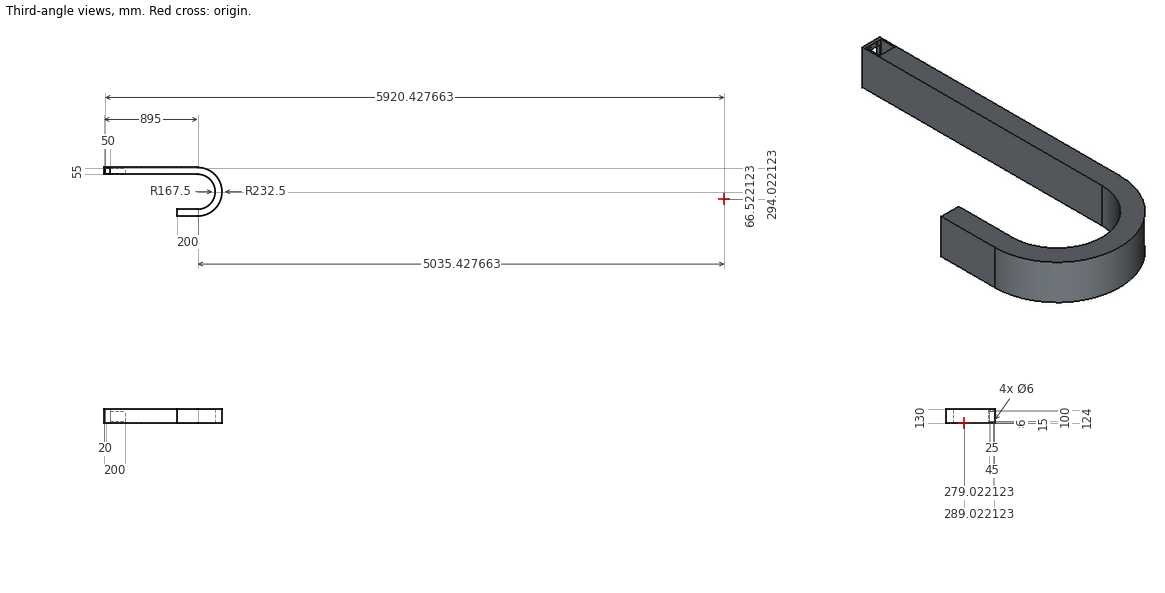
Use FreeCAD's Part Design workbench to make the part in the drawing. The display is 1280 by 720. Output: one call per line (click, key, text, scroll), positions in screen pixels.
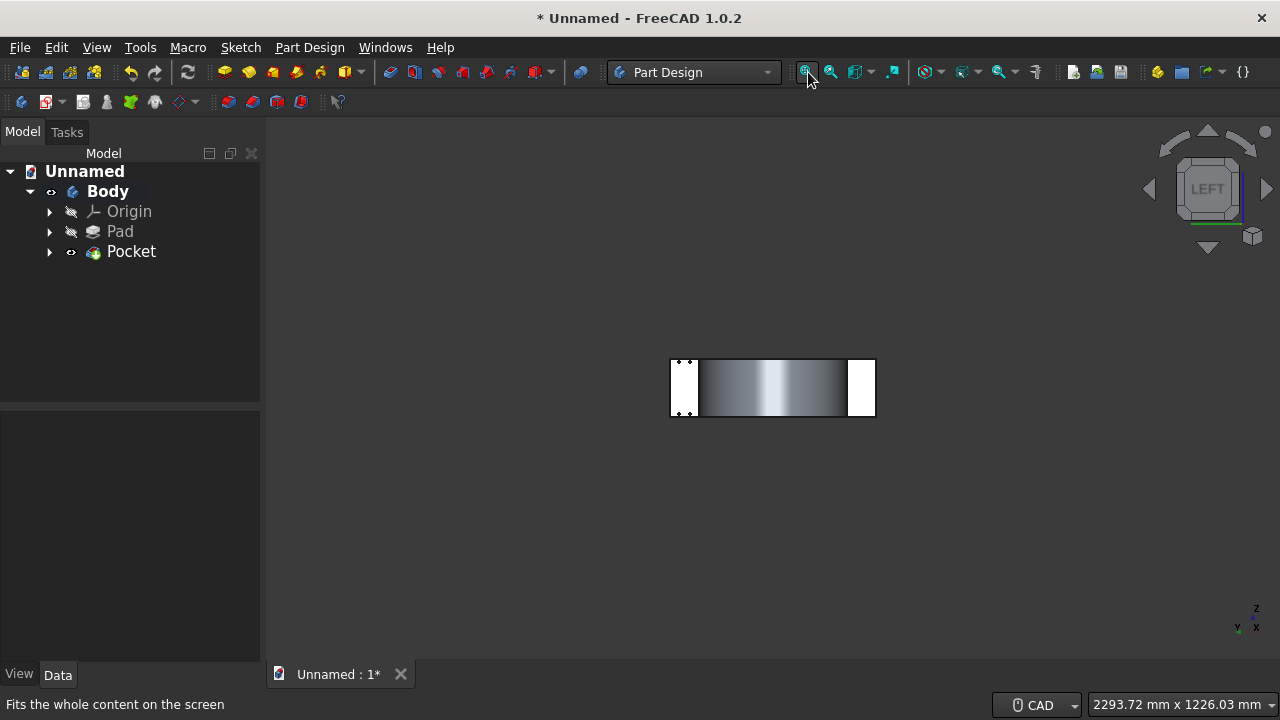
key(0)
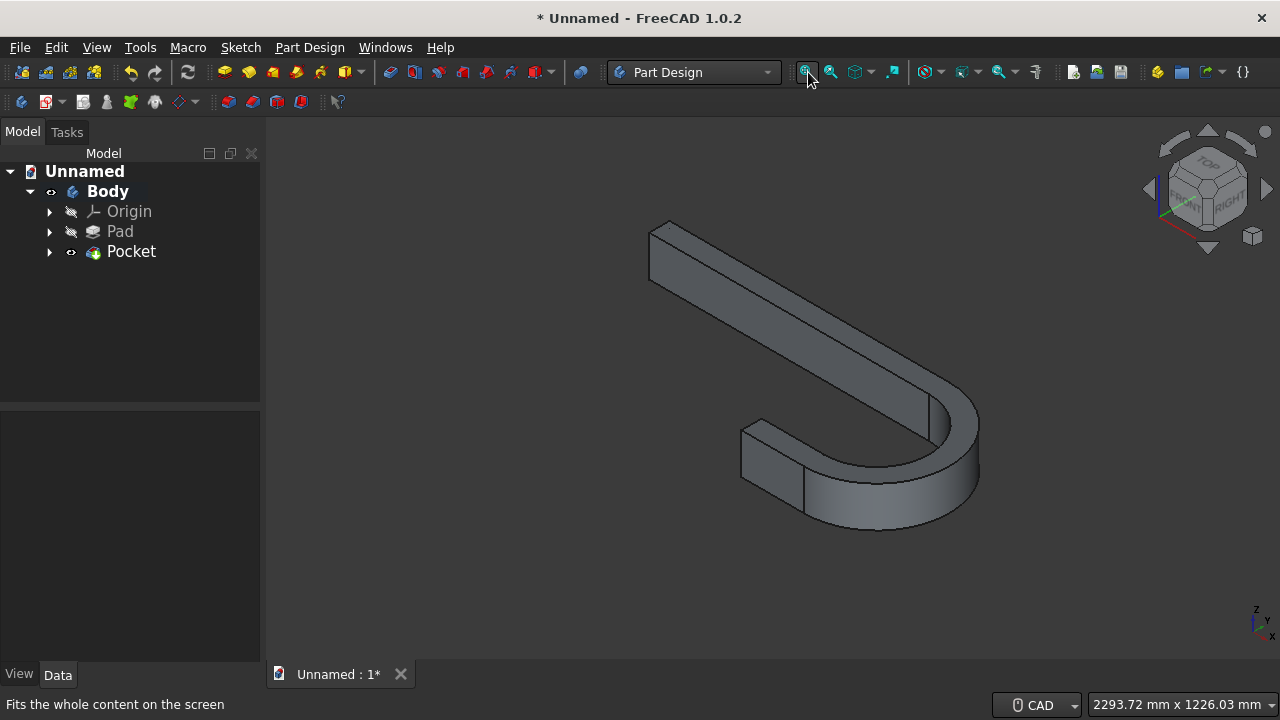
click(936, 386)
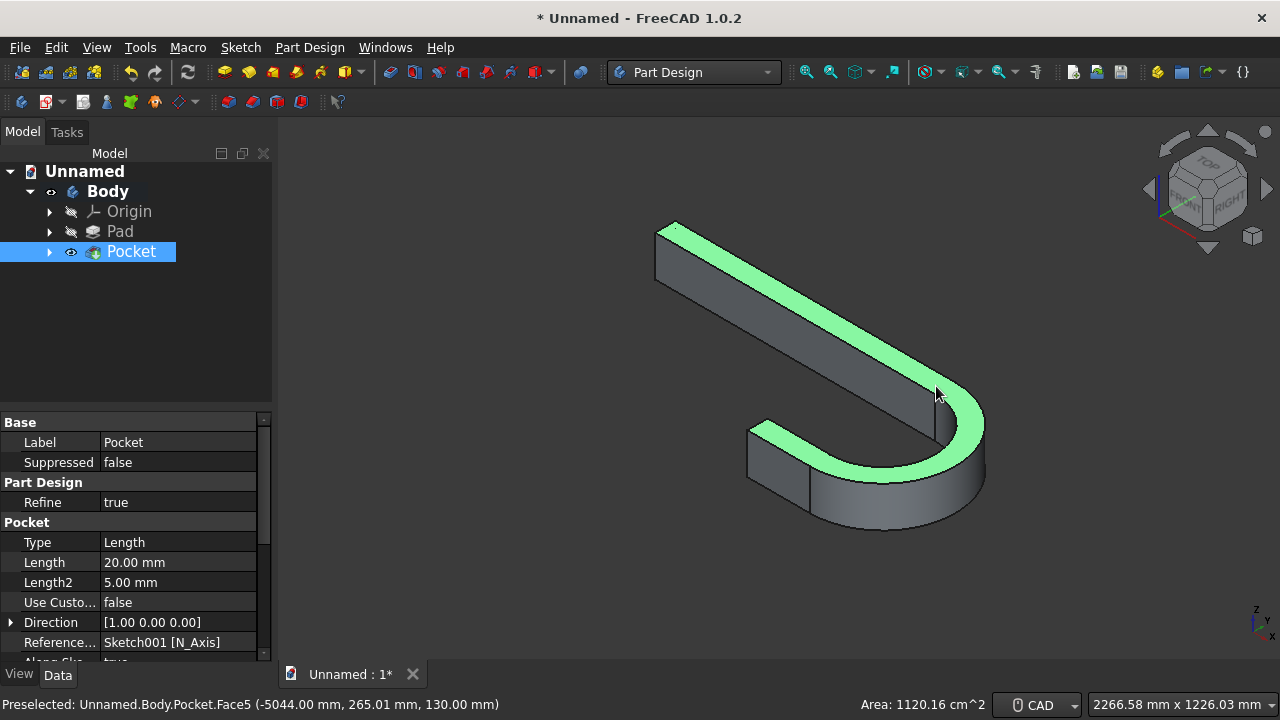
click(46, 102)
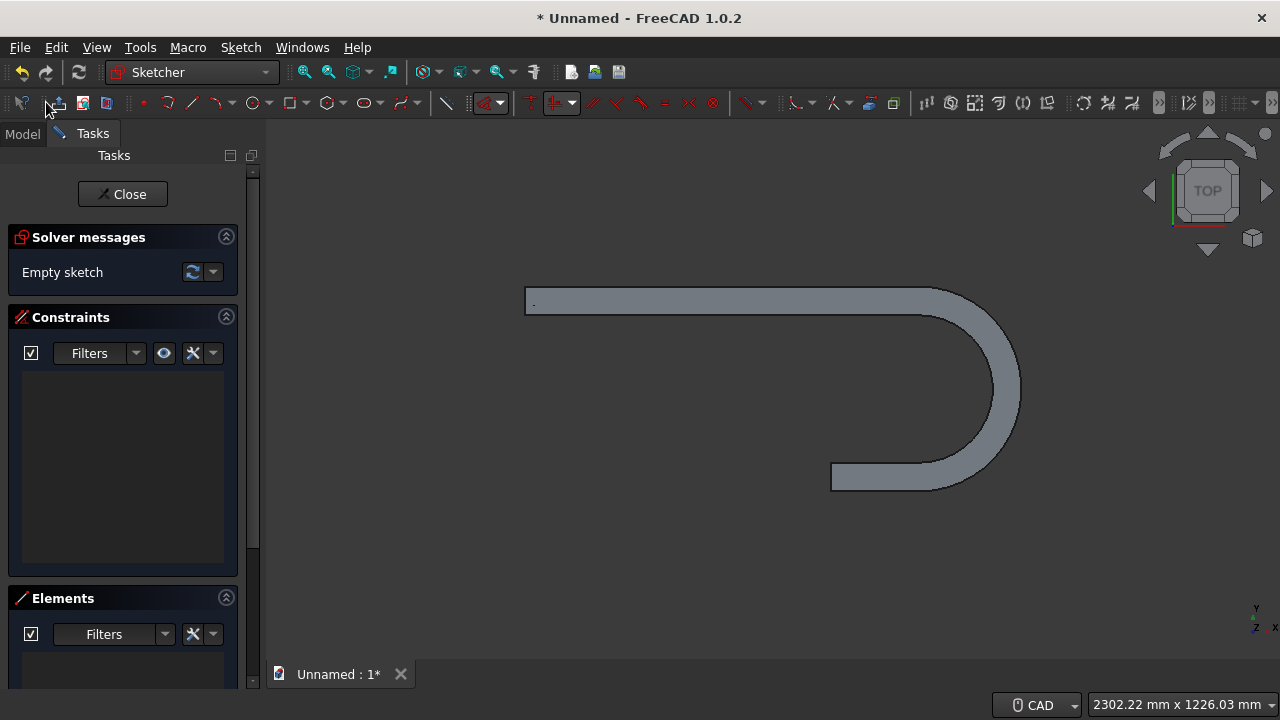
scroll(527, 294, up, 13)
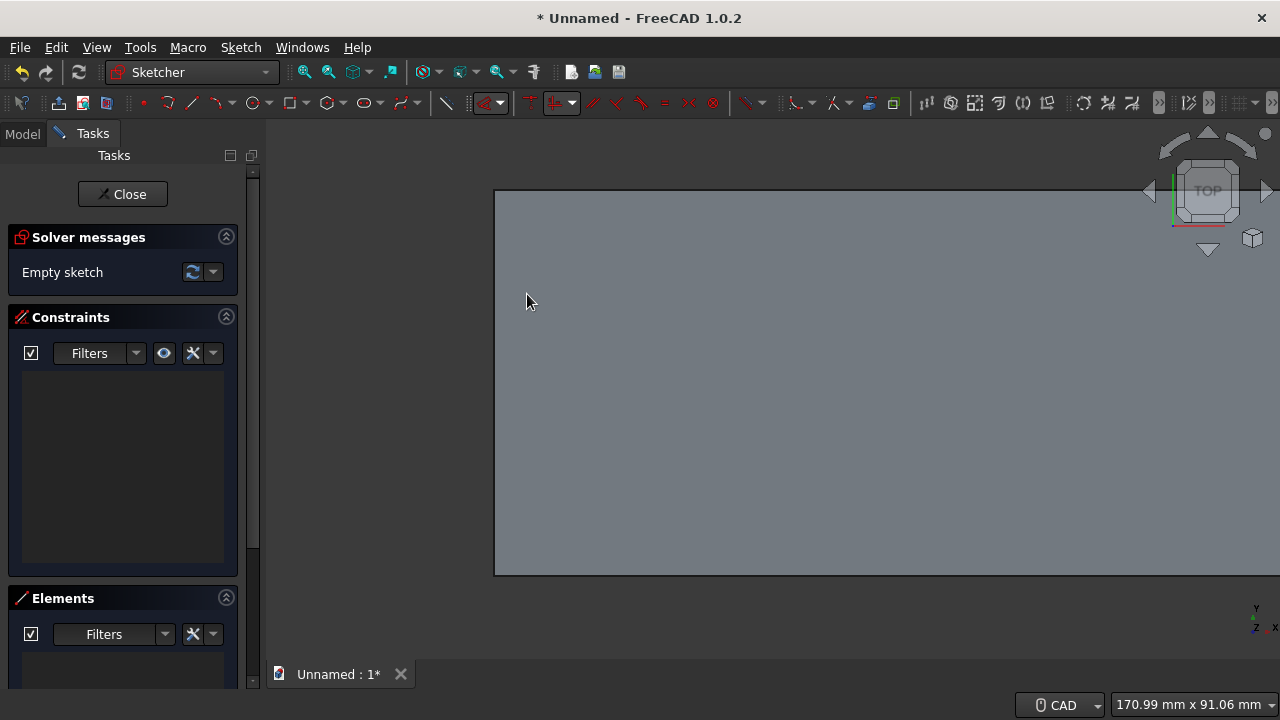
key(g)
key(r)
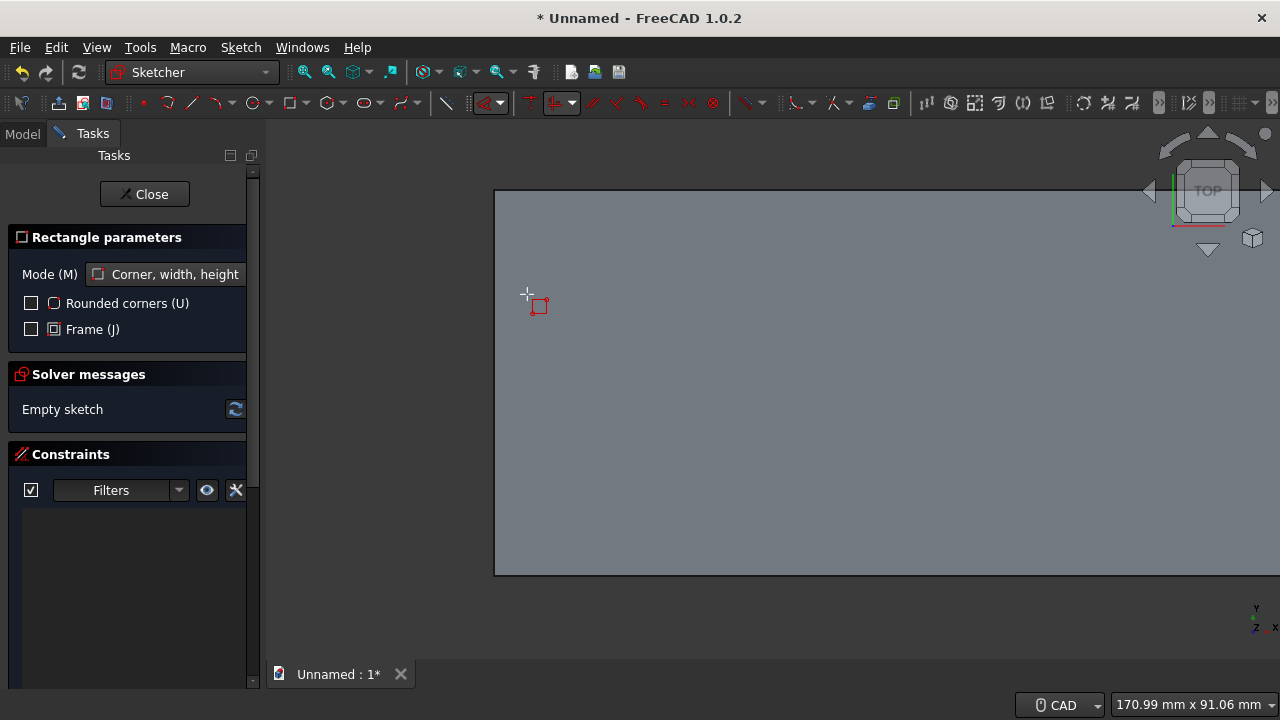
click(554, 220)
move(850, 546)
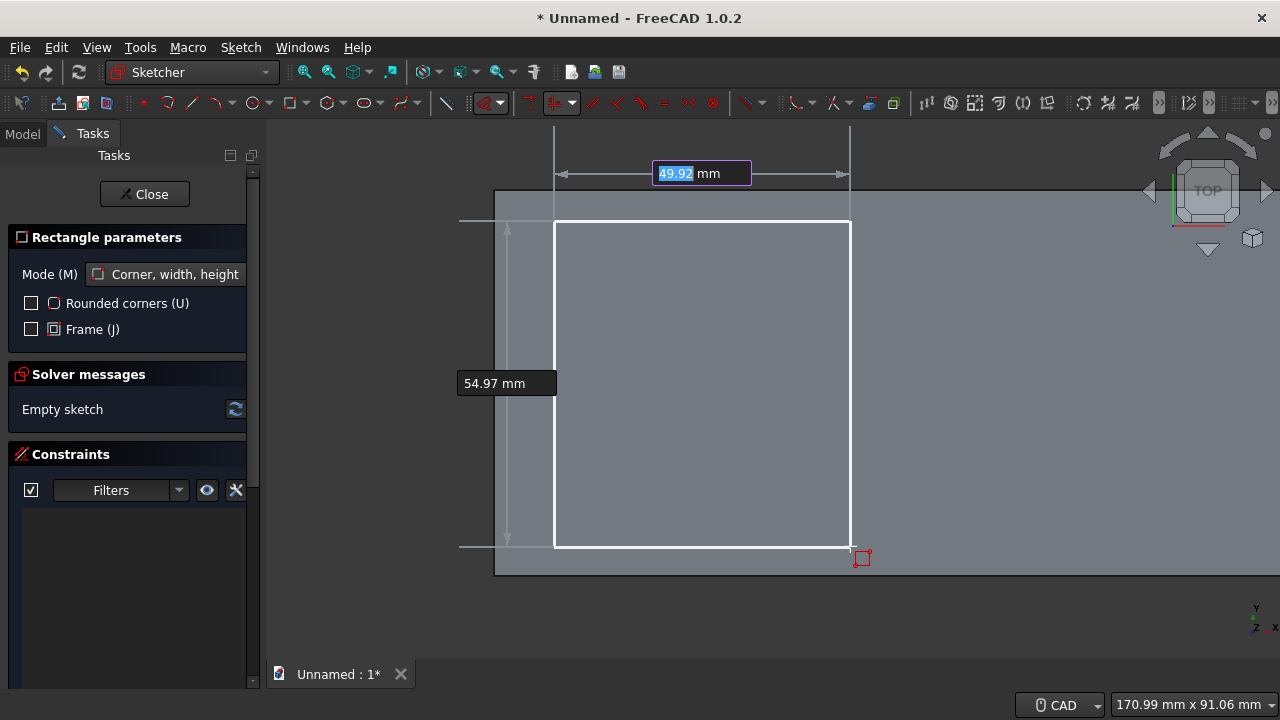
text(50)
key(Tab)
text(55)
key(Return)
key(Escape)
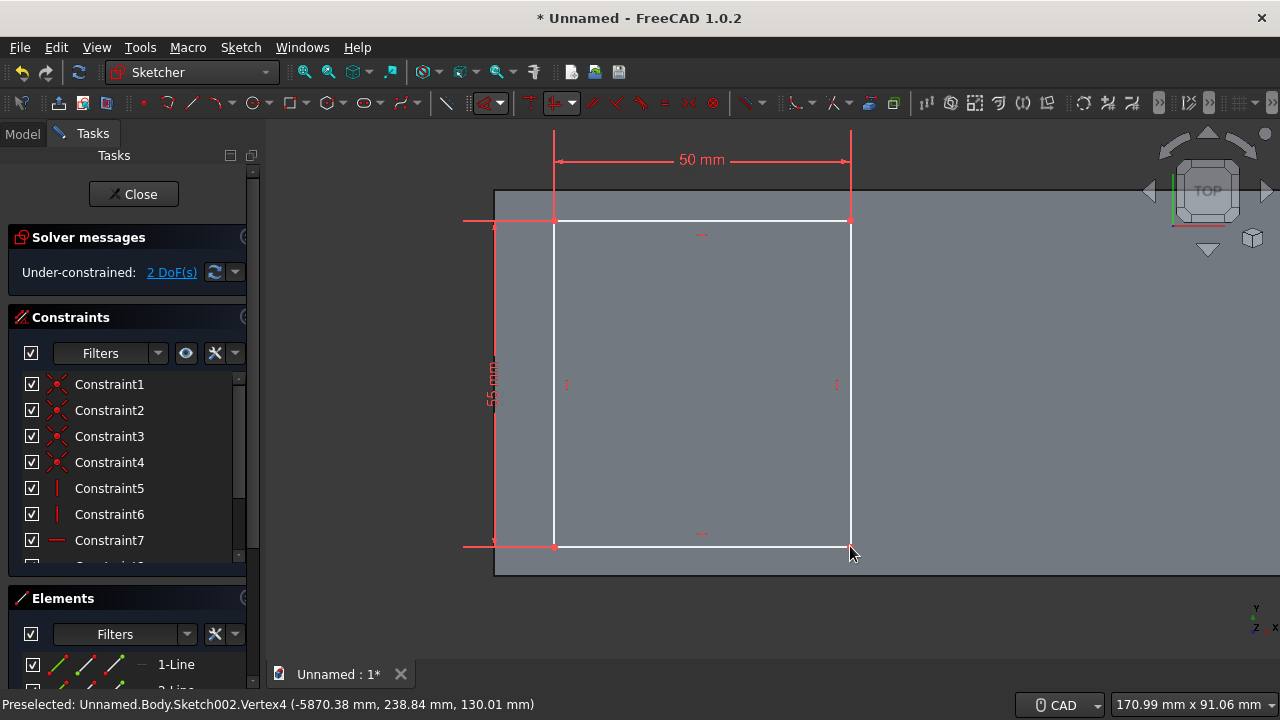
click(554, 221)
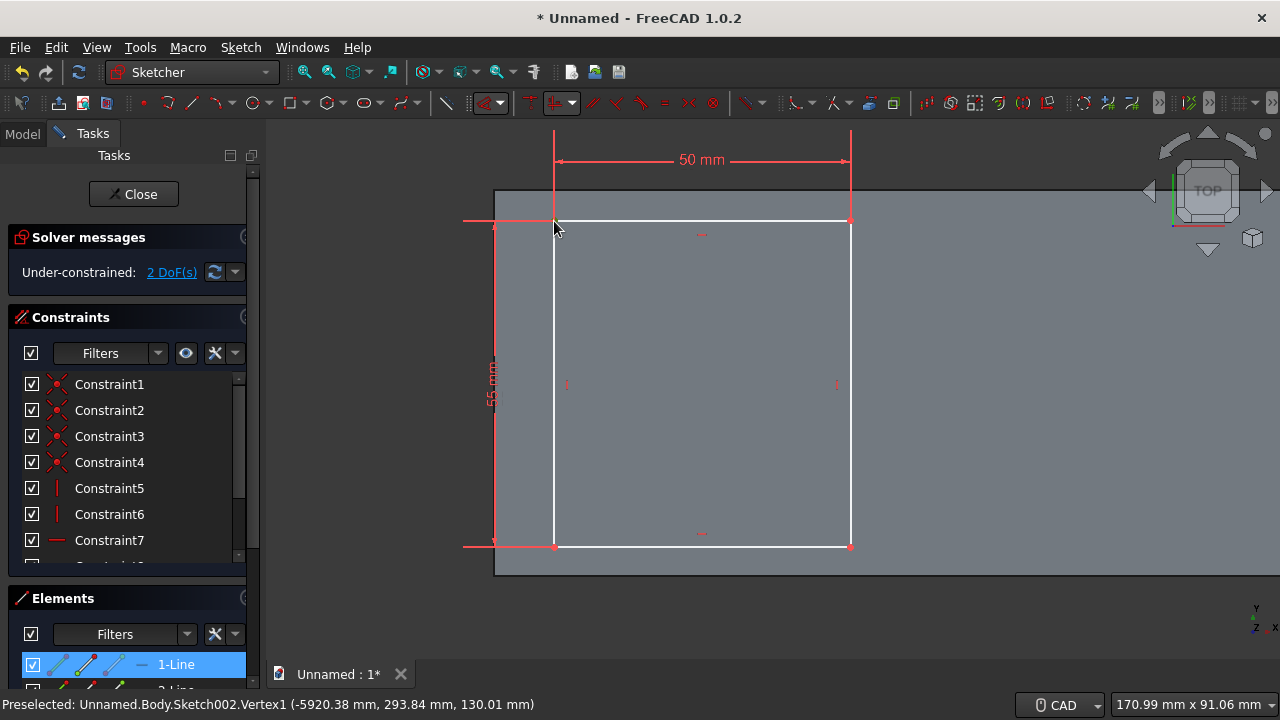
key(i)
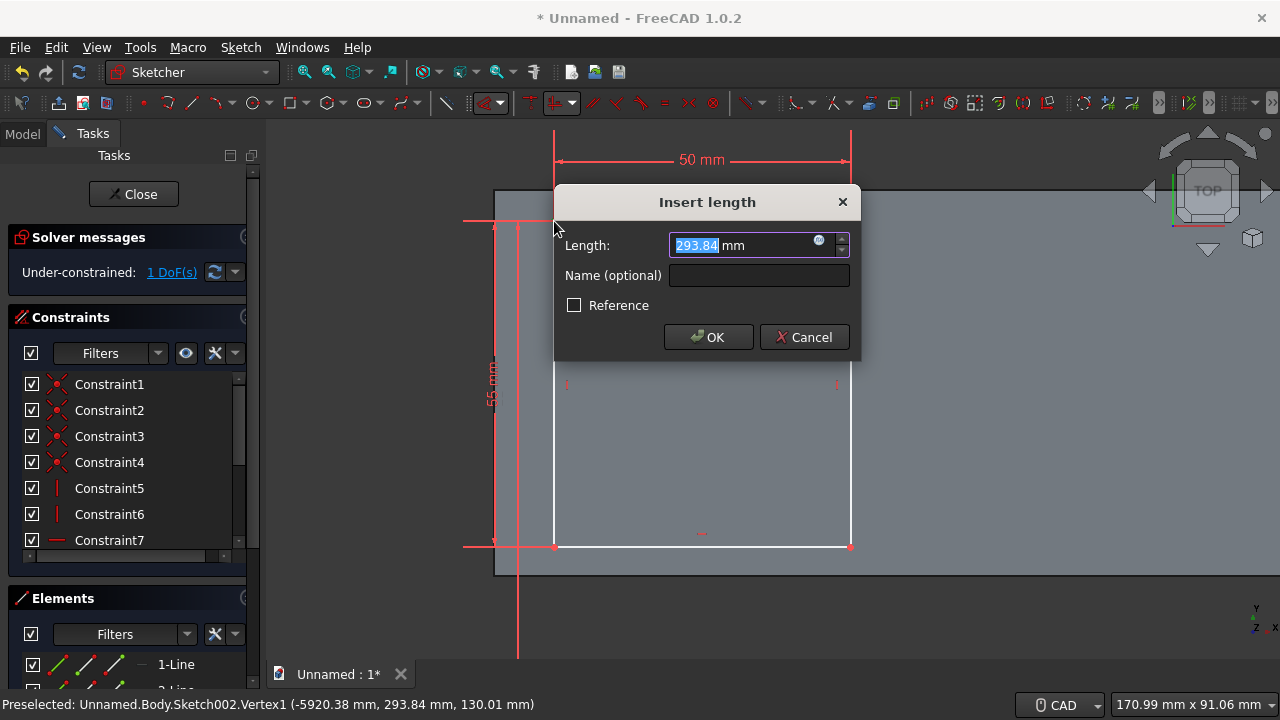
text(294.022123)
key(Return)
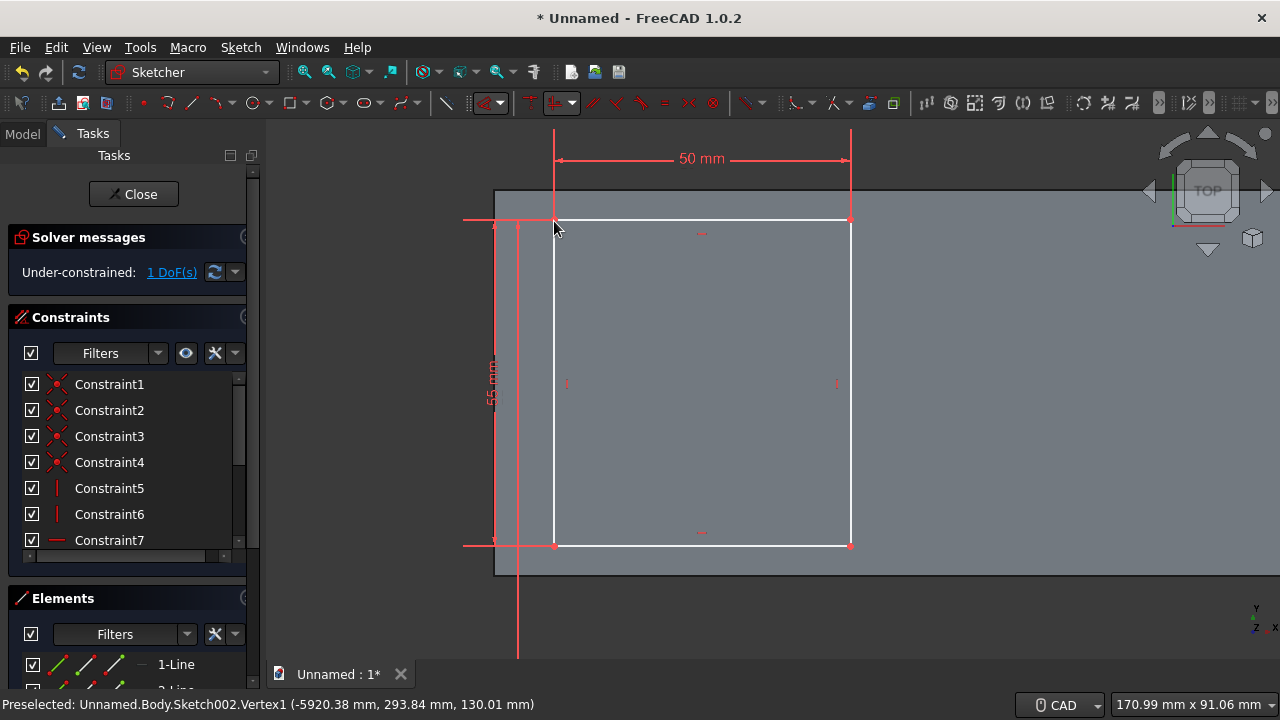
click(554, 220)